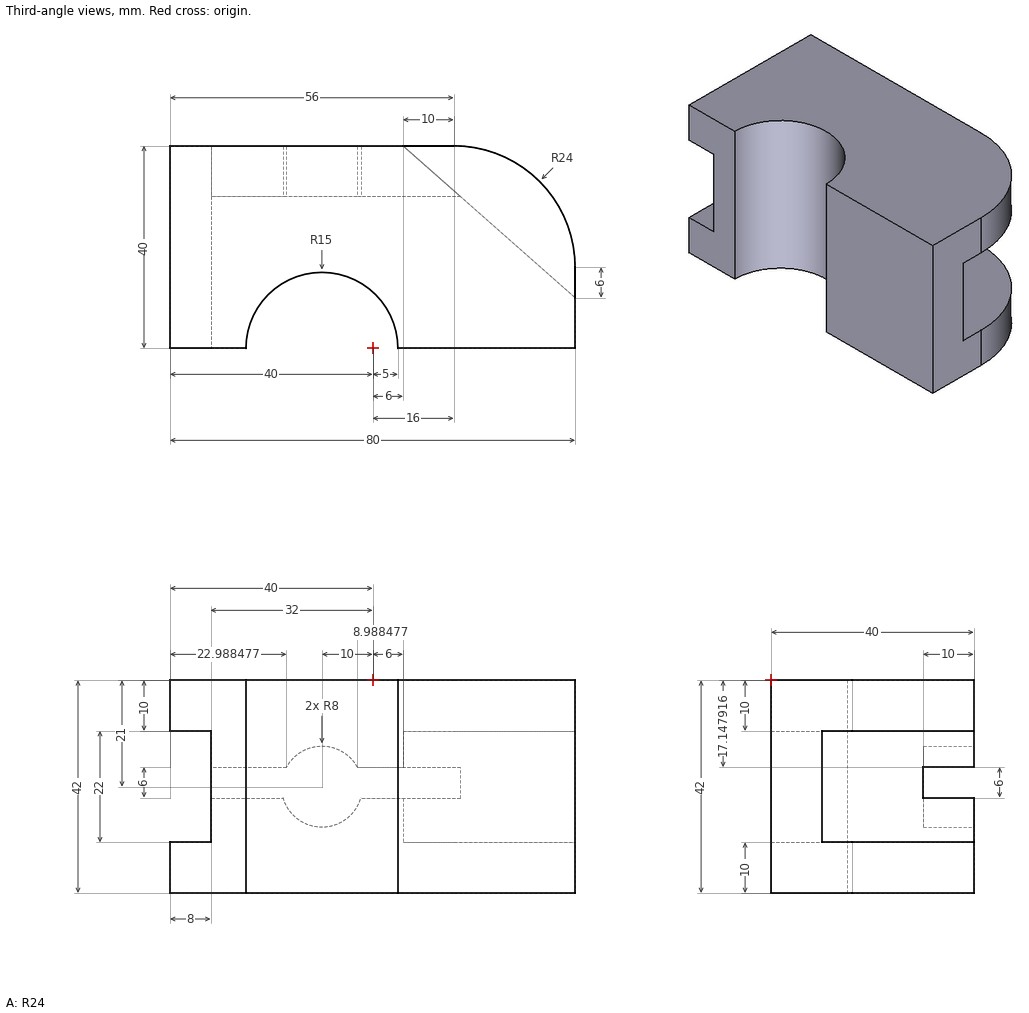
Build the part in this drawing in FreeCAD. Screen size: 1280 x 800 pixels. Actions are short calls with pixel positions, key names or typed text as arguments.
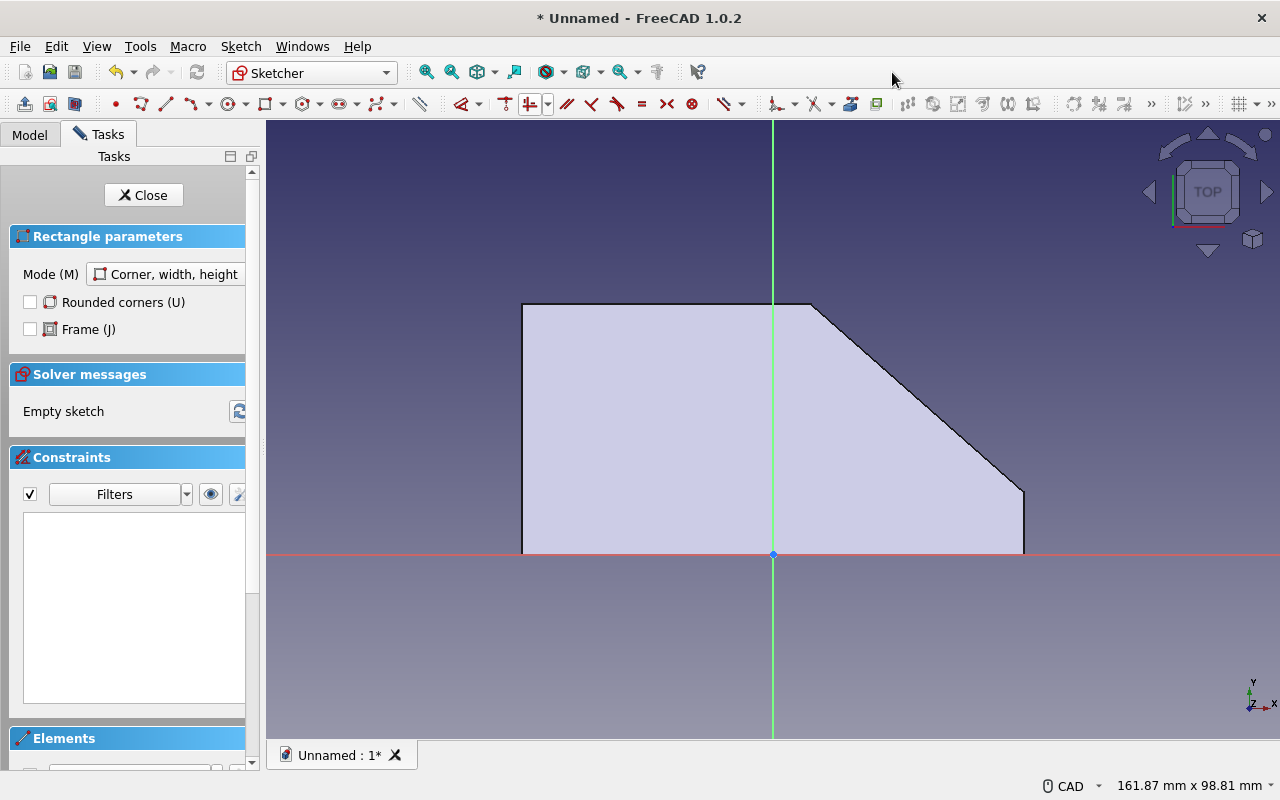
click(522, 304)
click(1024, 555)
key(Escape)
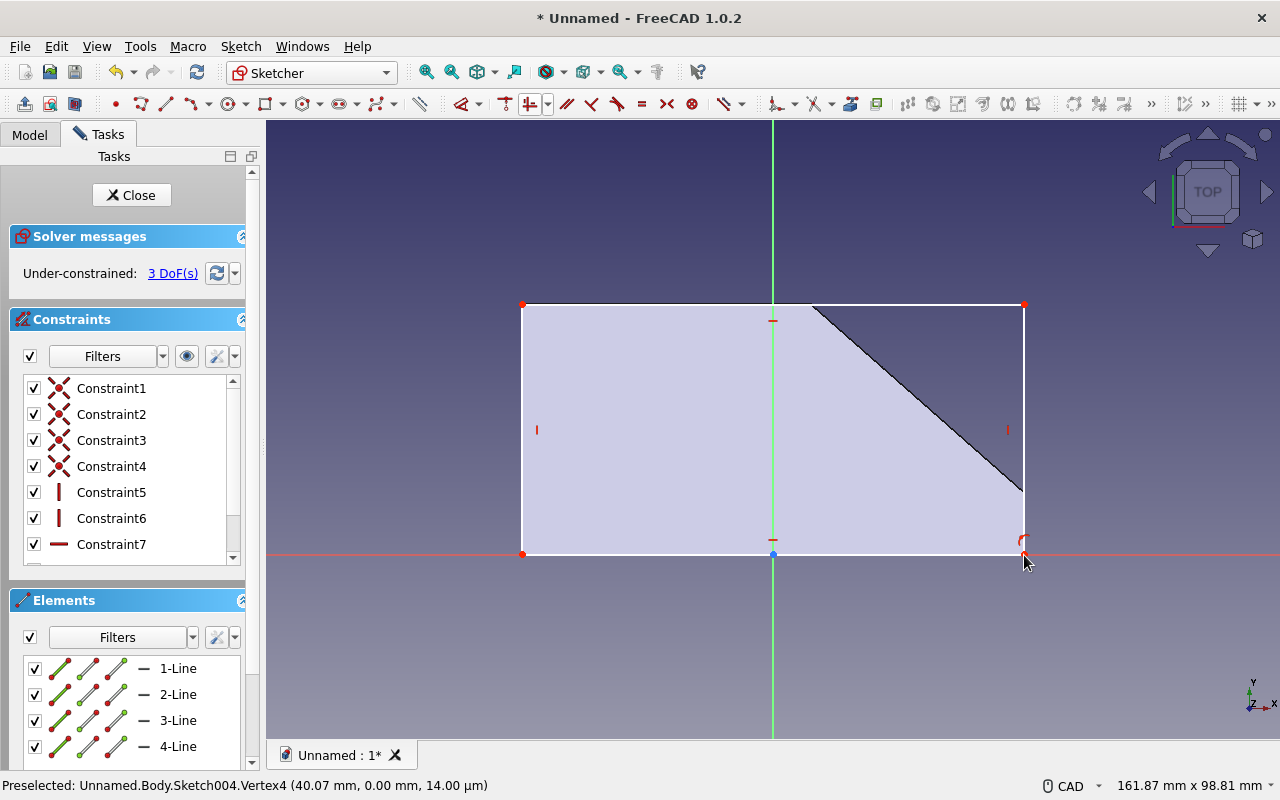
click(460, 104)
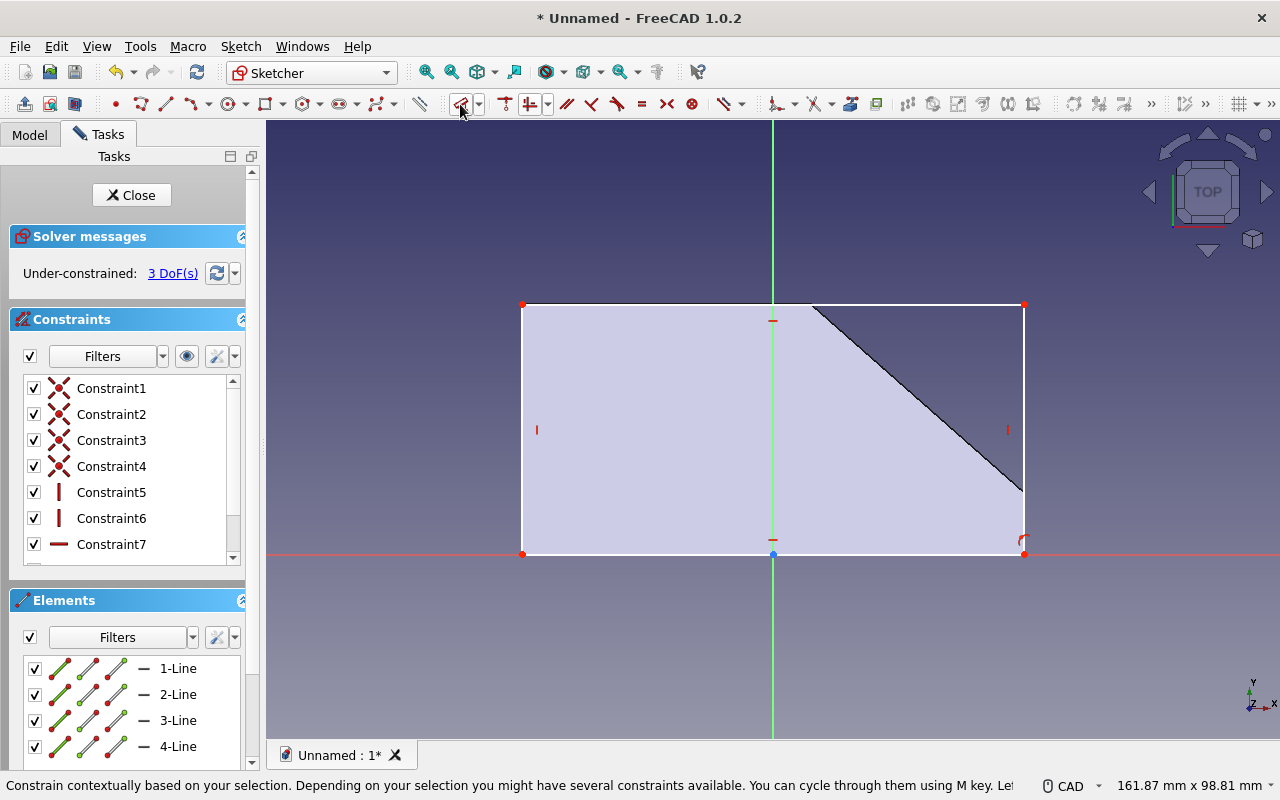
click(522, 380)
click(488, 430)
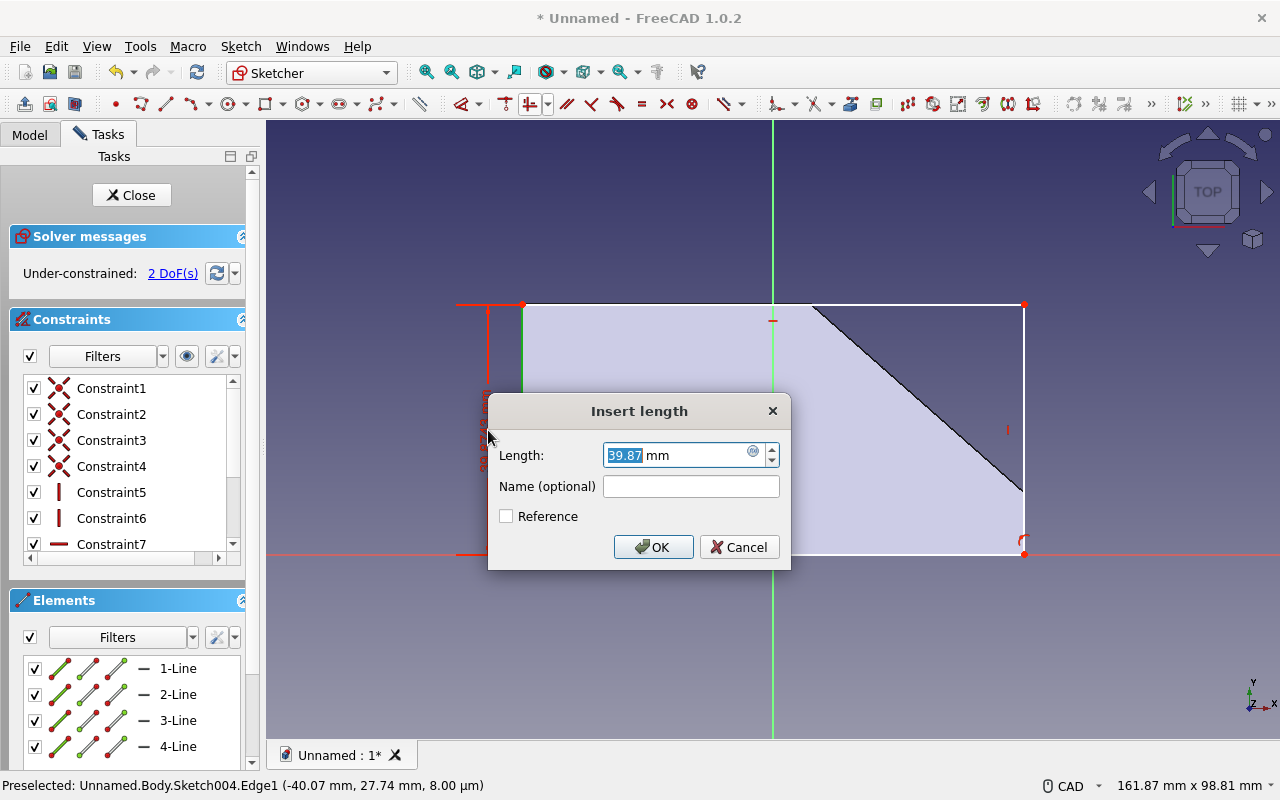
text(40)
key(Return)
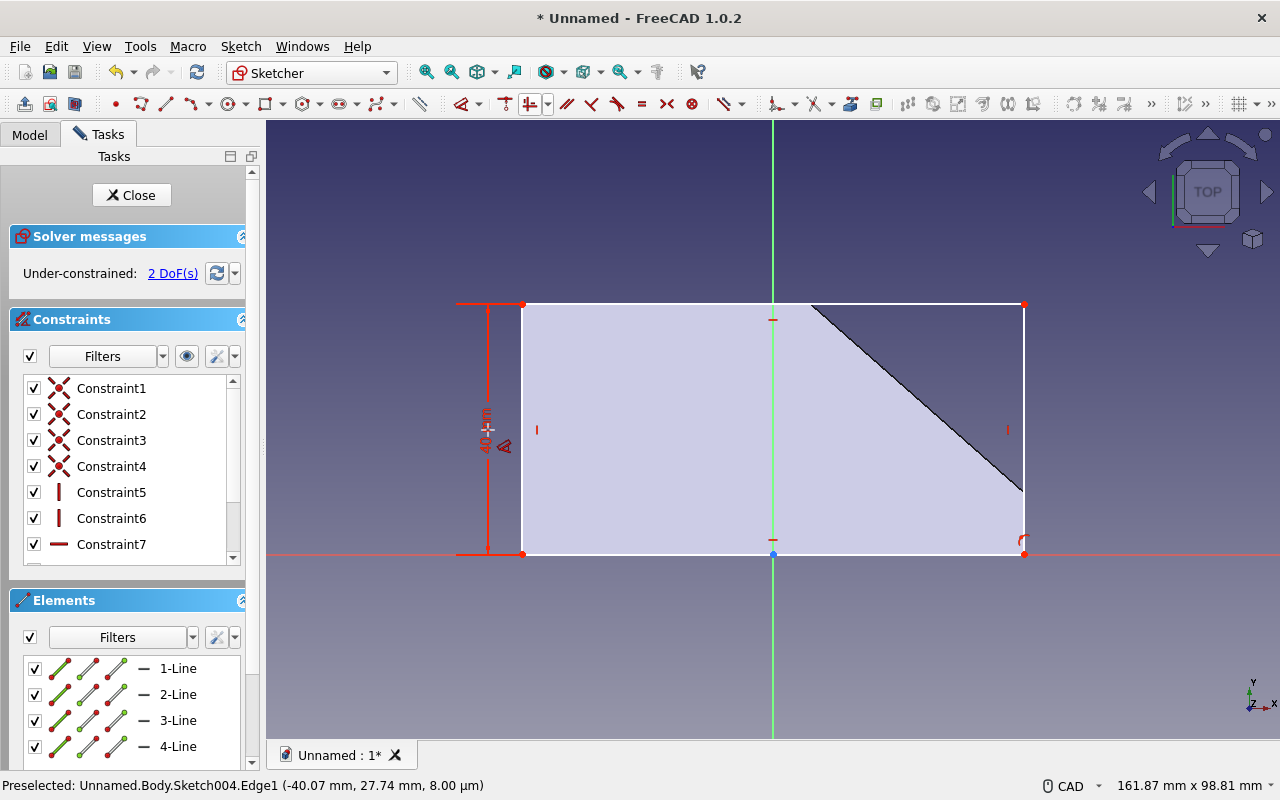
click(673, 555)
click(658, 589)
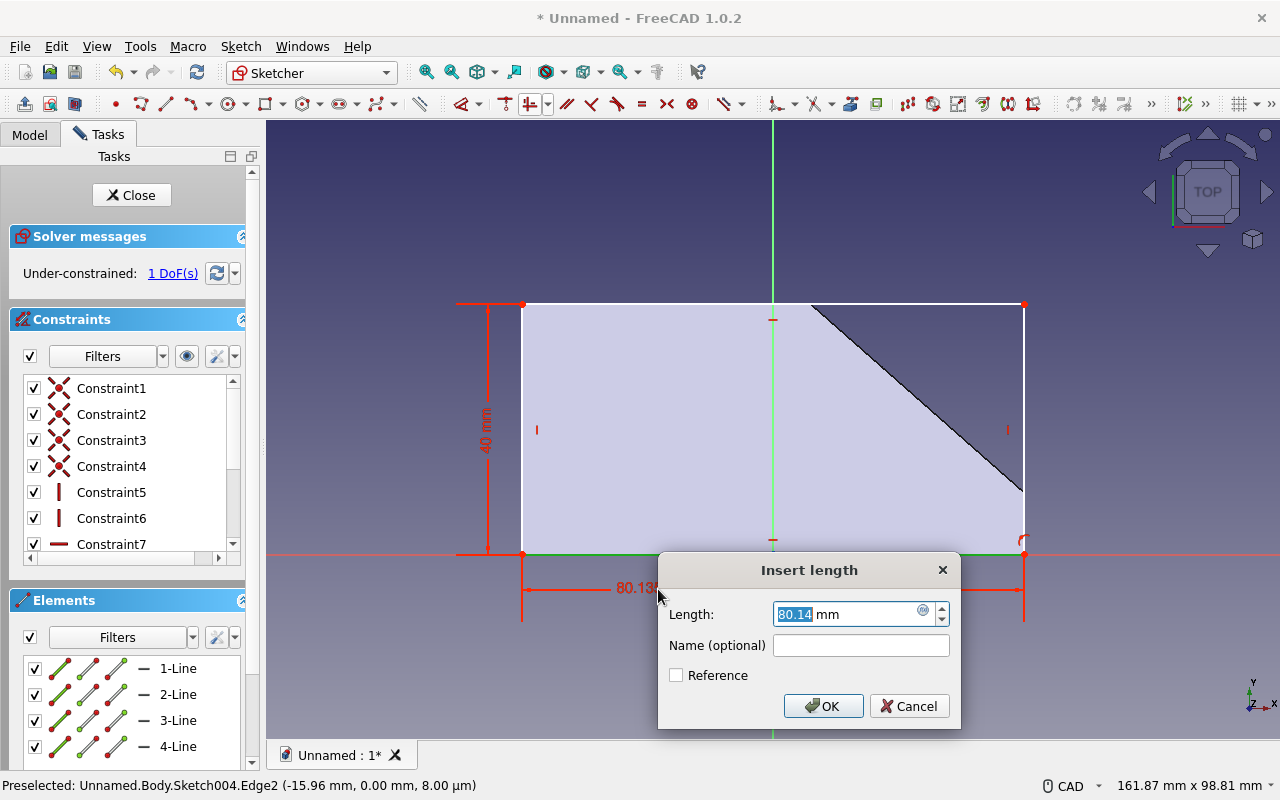
text(80)
key(Return)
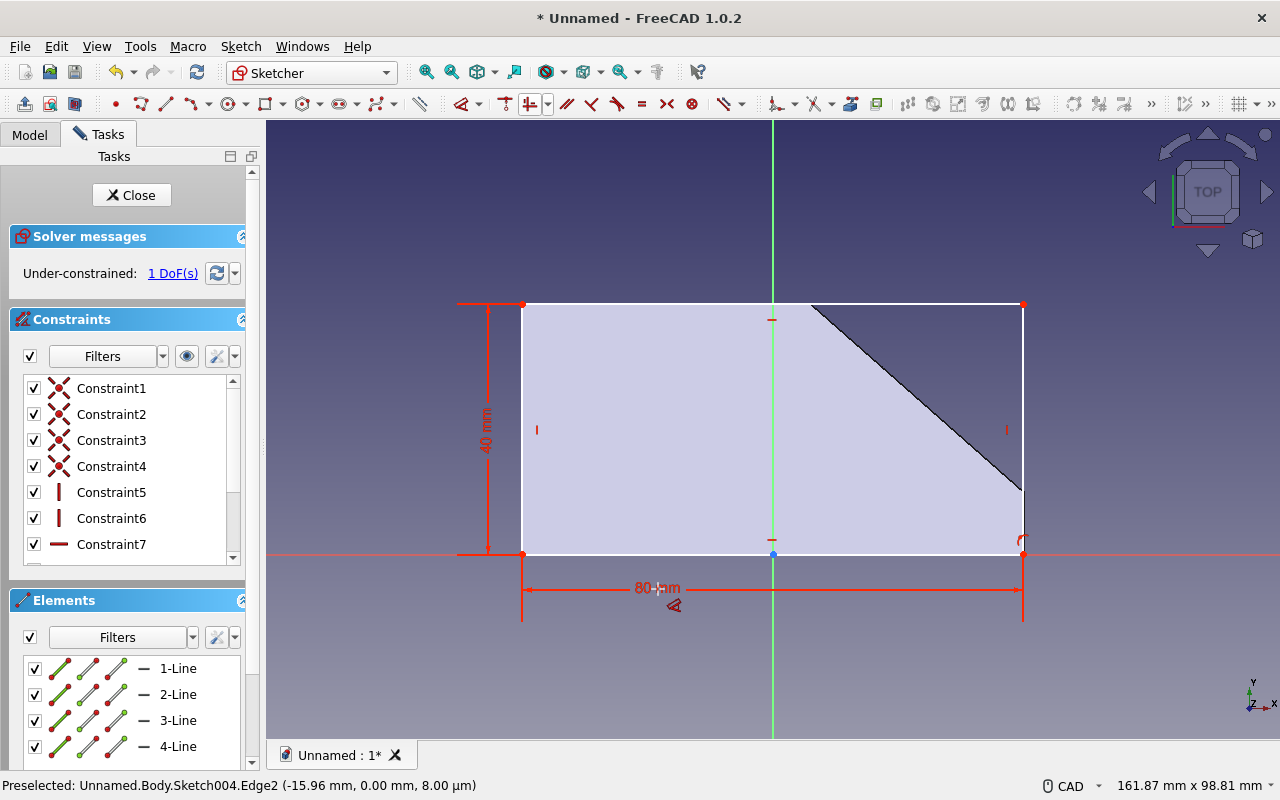
click(522, 304)
click(560, 589)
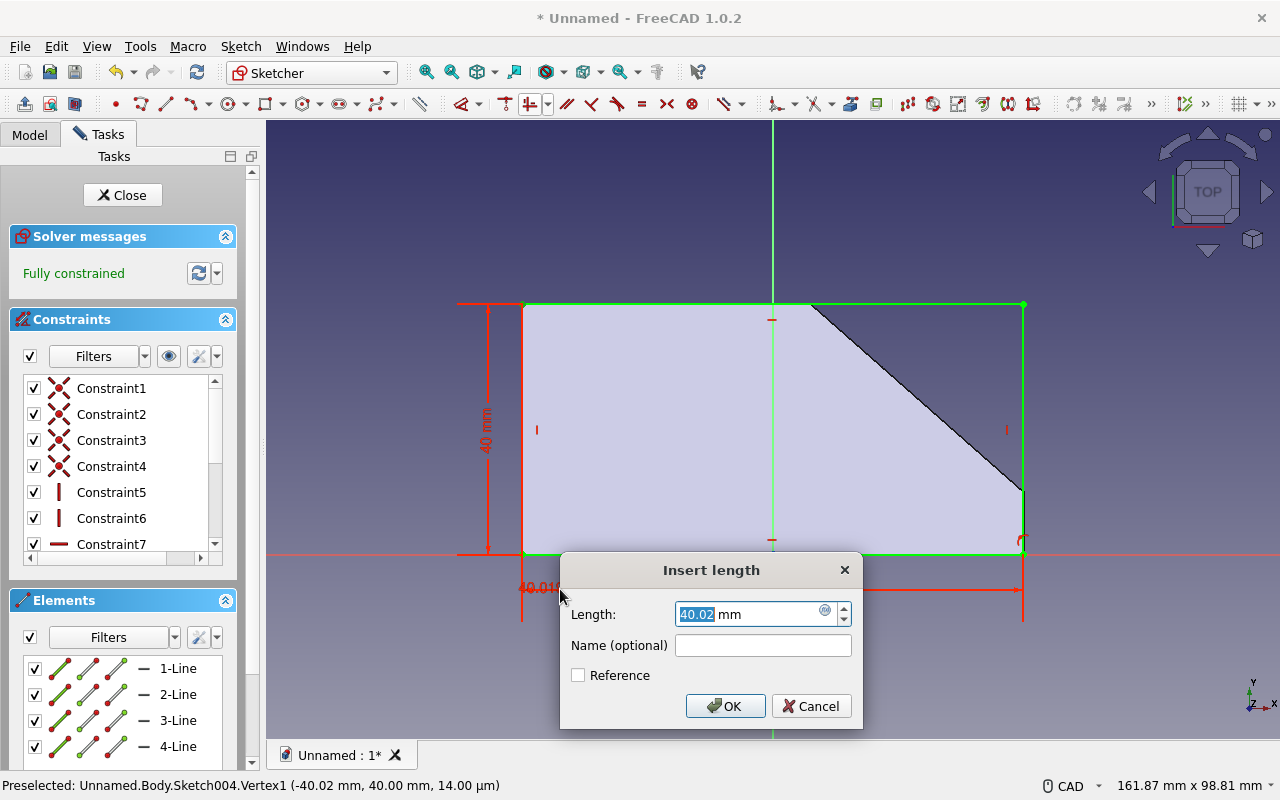
text(40)
key(Return)
key(Escape)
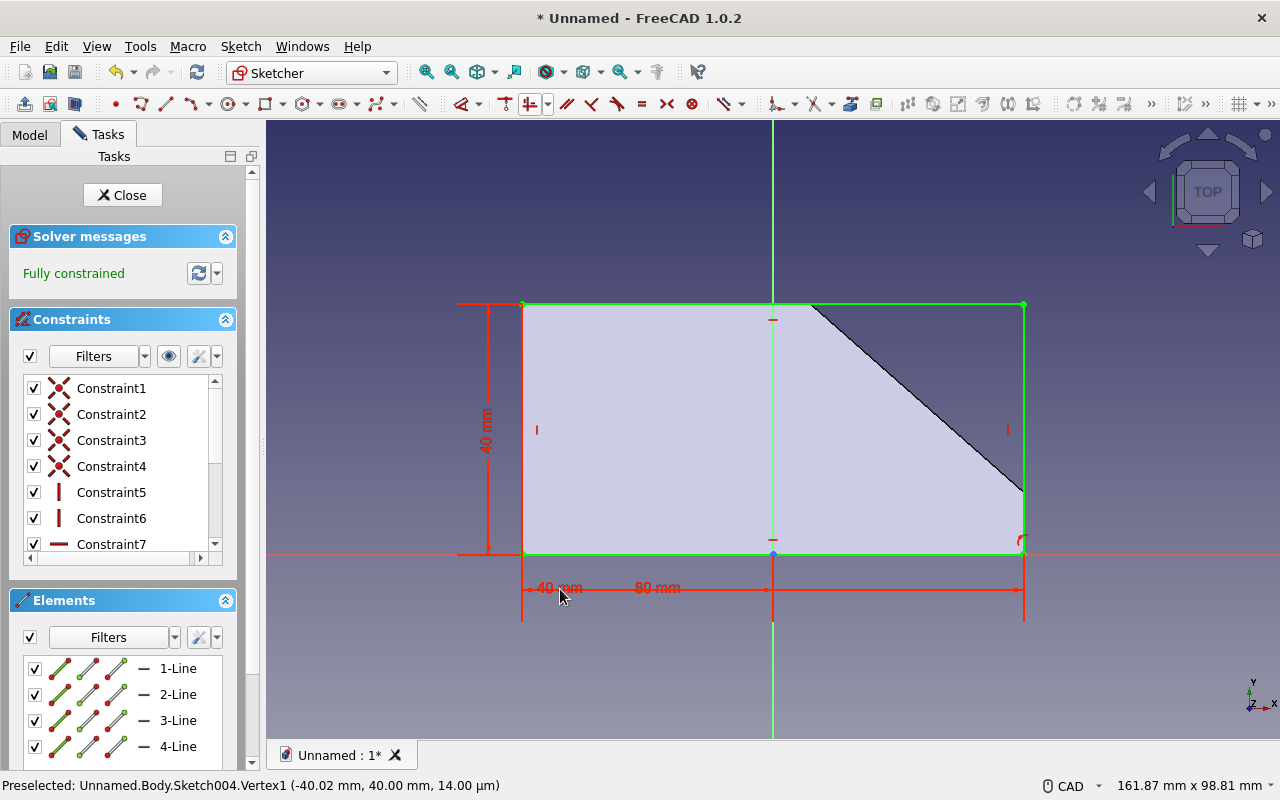
click(123, 195)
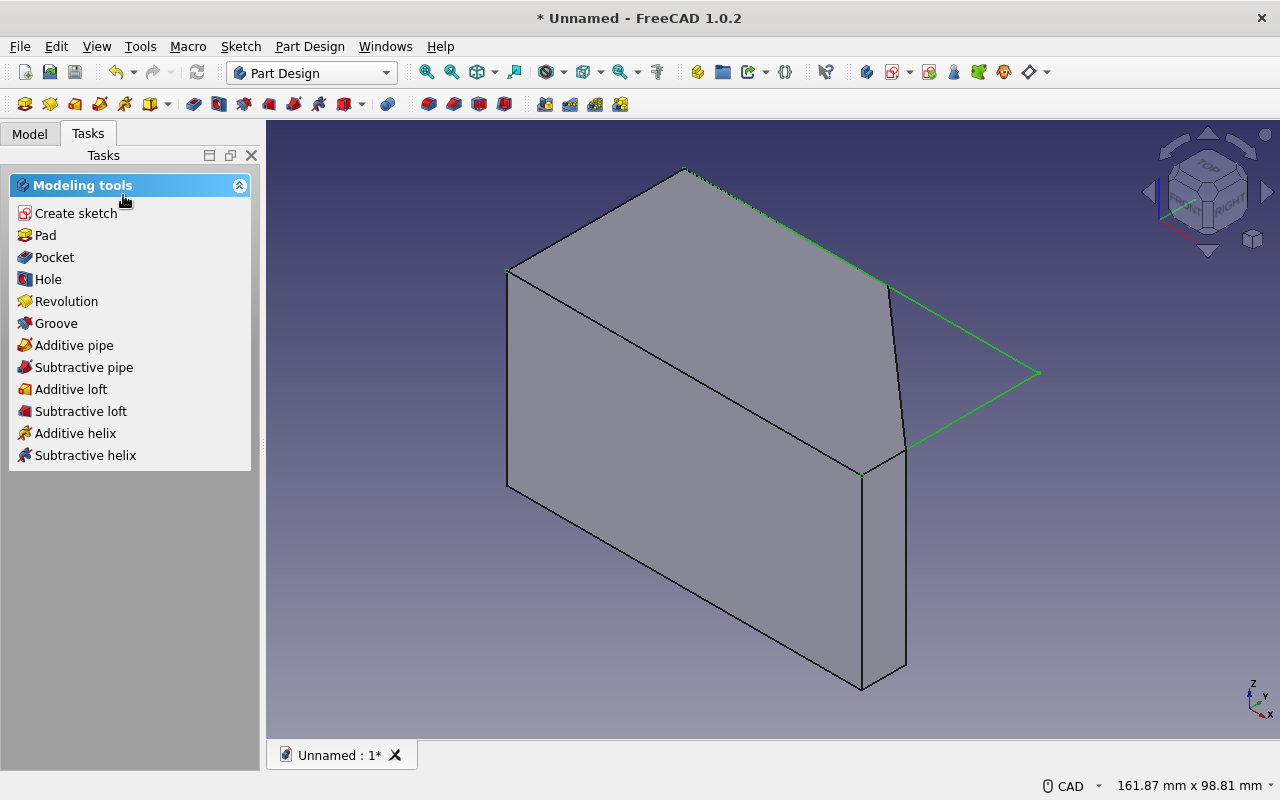
click(25, 104)